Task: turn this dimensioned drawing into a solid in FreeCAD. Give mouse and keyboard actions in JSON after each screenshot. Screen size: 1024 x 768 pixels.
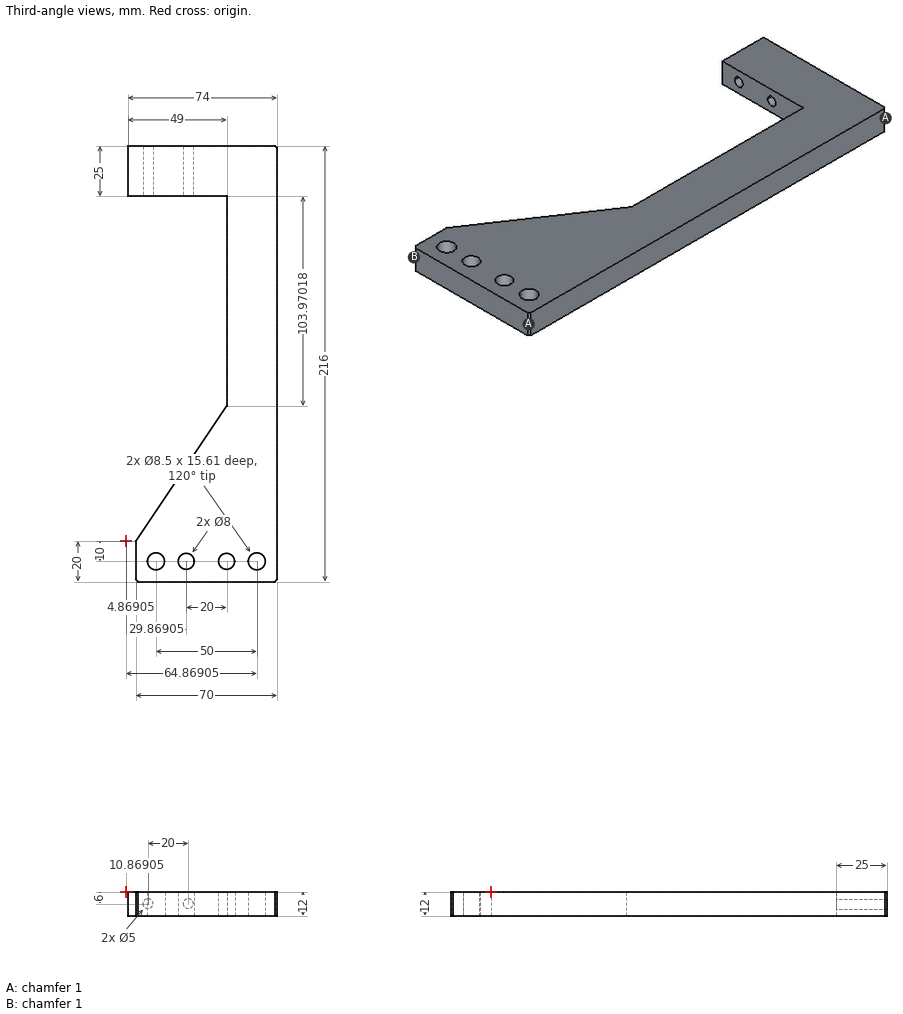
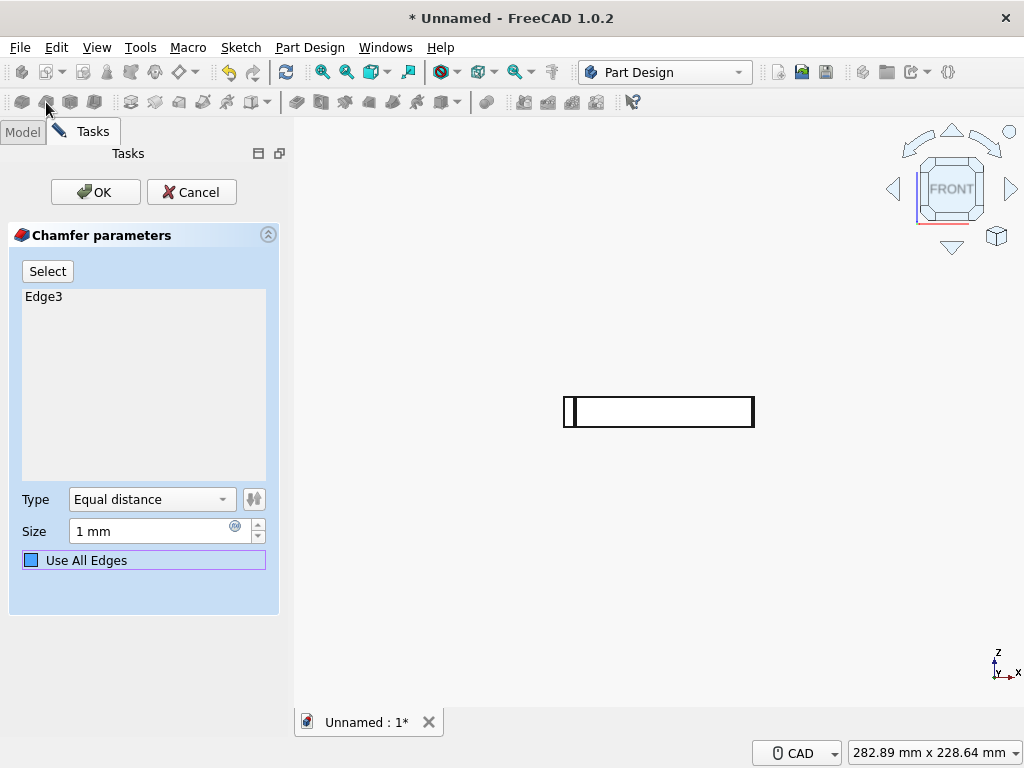
{"action": "left_click", "coordinate": [96, 192]}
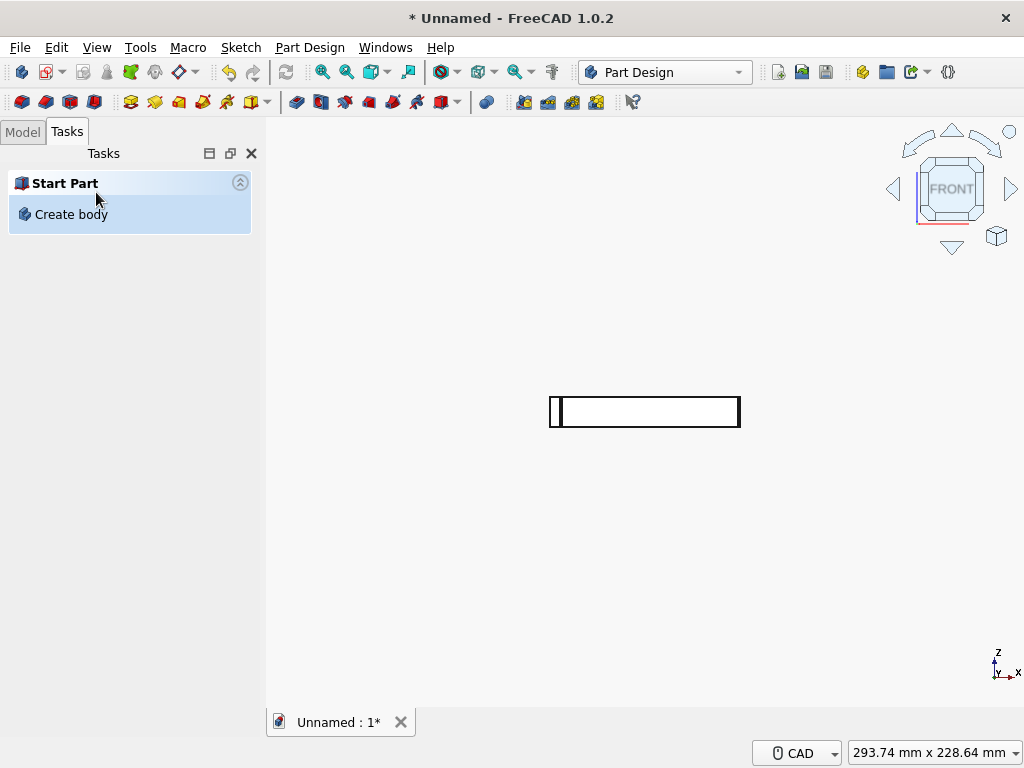
{"action": "key", "text": "0"}